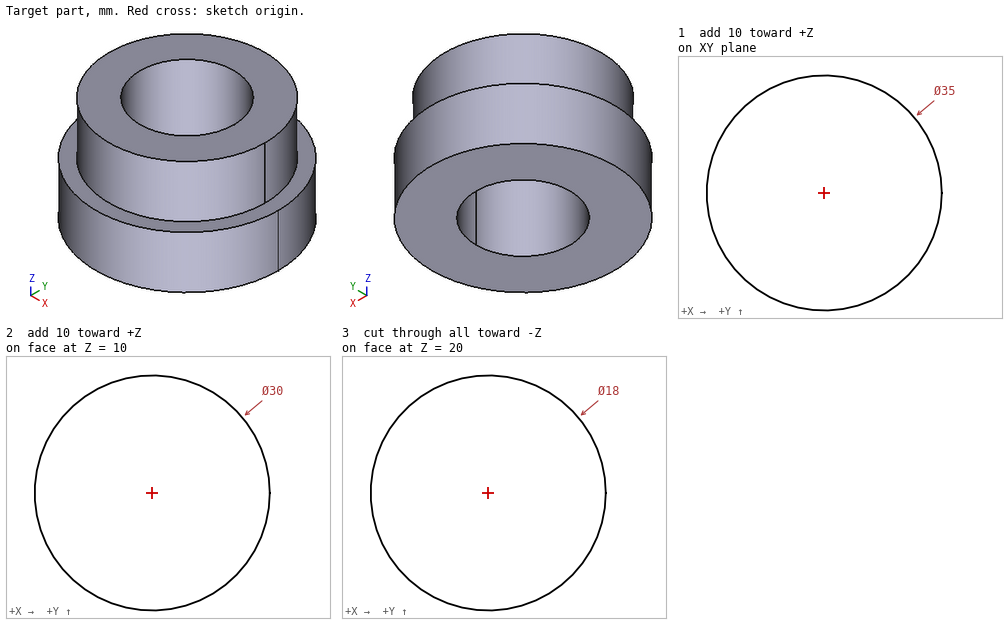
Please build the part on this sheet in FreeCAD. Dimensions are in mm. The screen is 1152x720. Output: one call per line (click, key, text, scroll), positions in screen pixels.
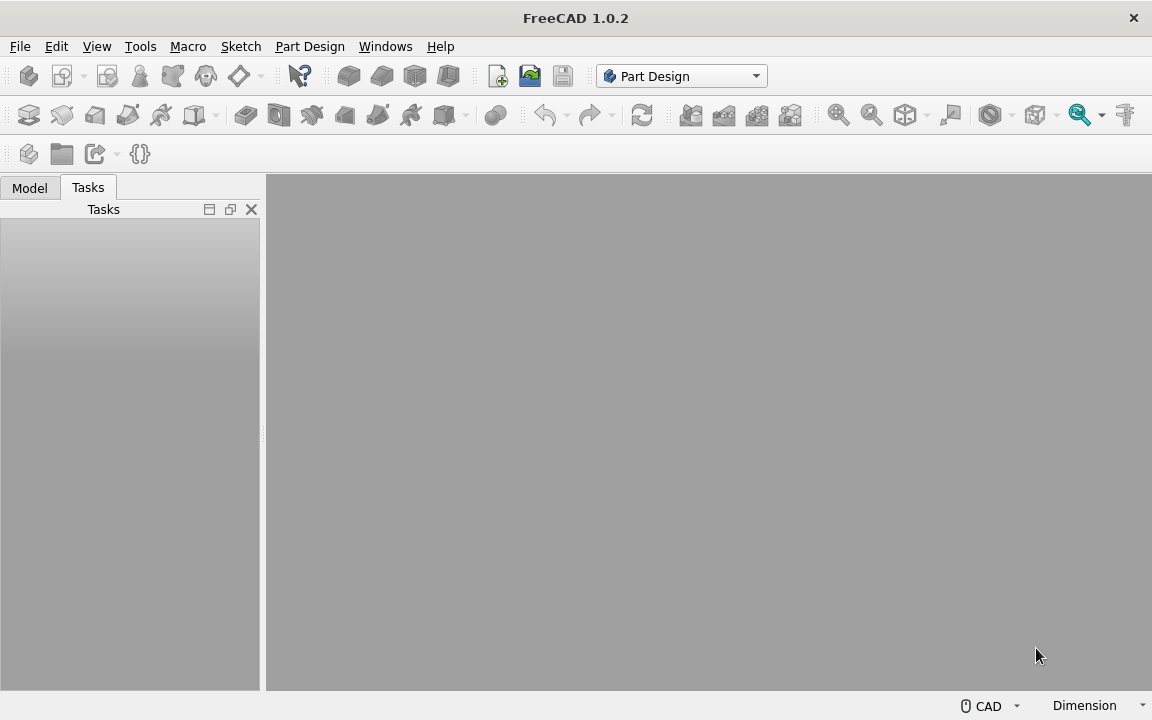
click(497, 76)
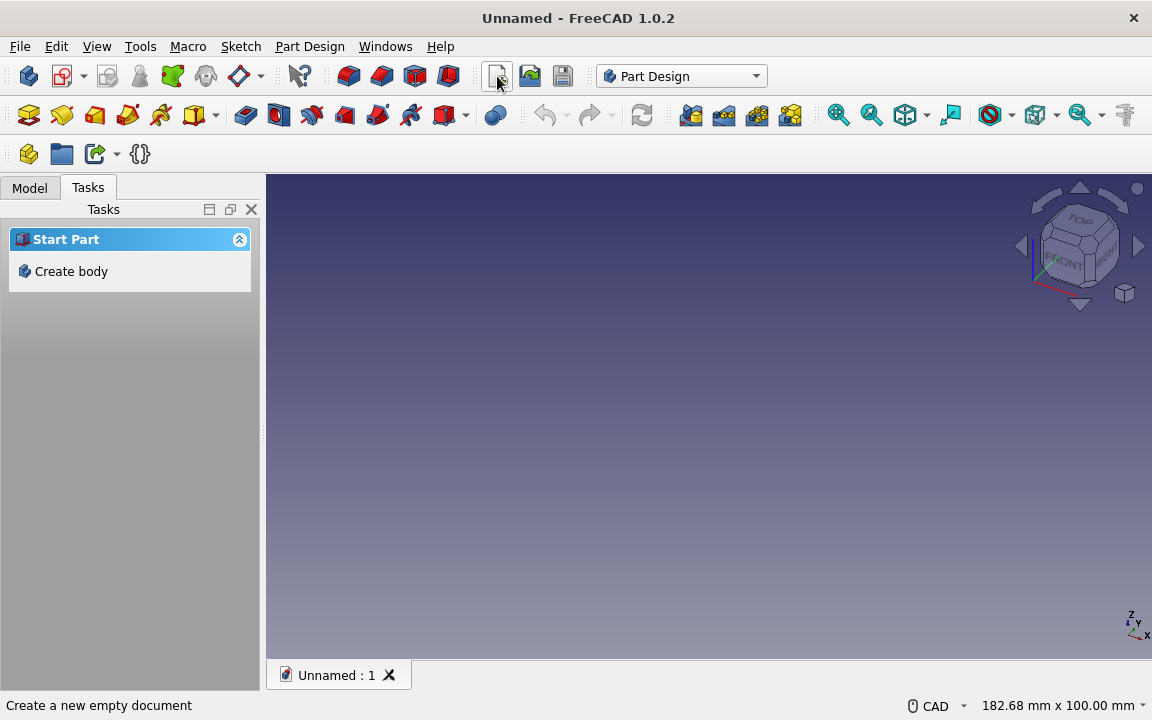
click(62, 76)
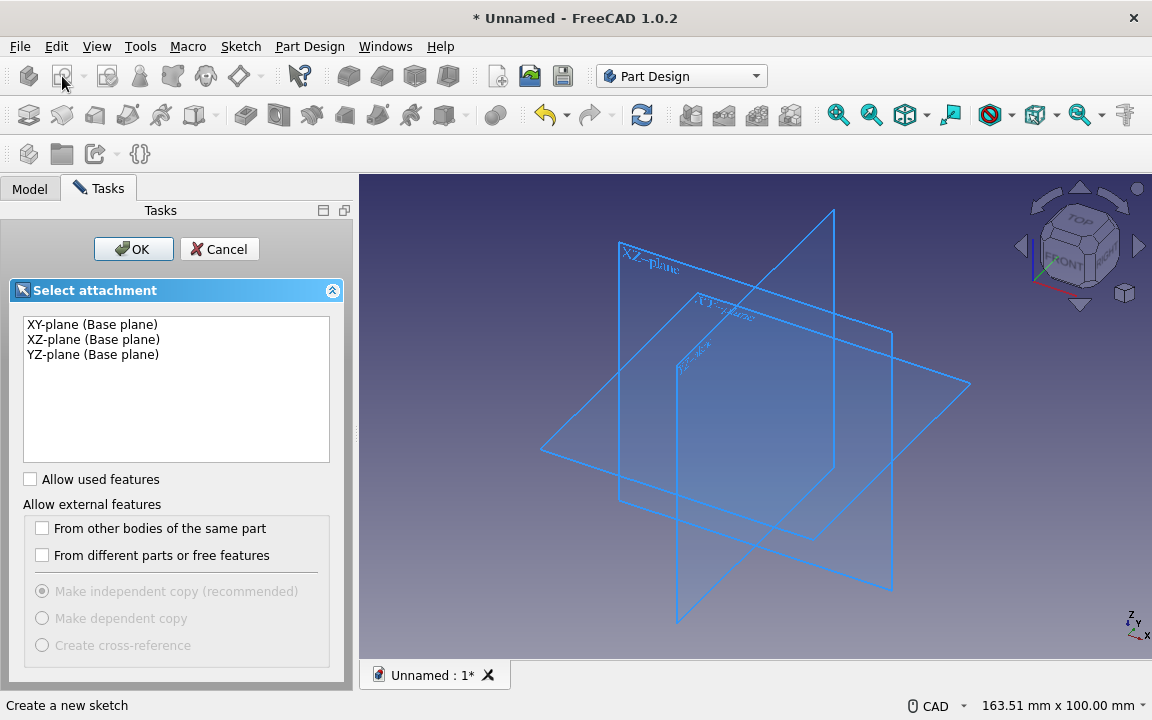
click(84, 324)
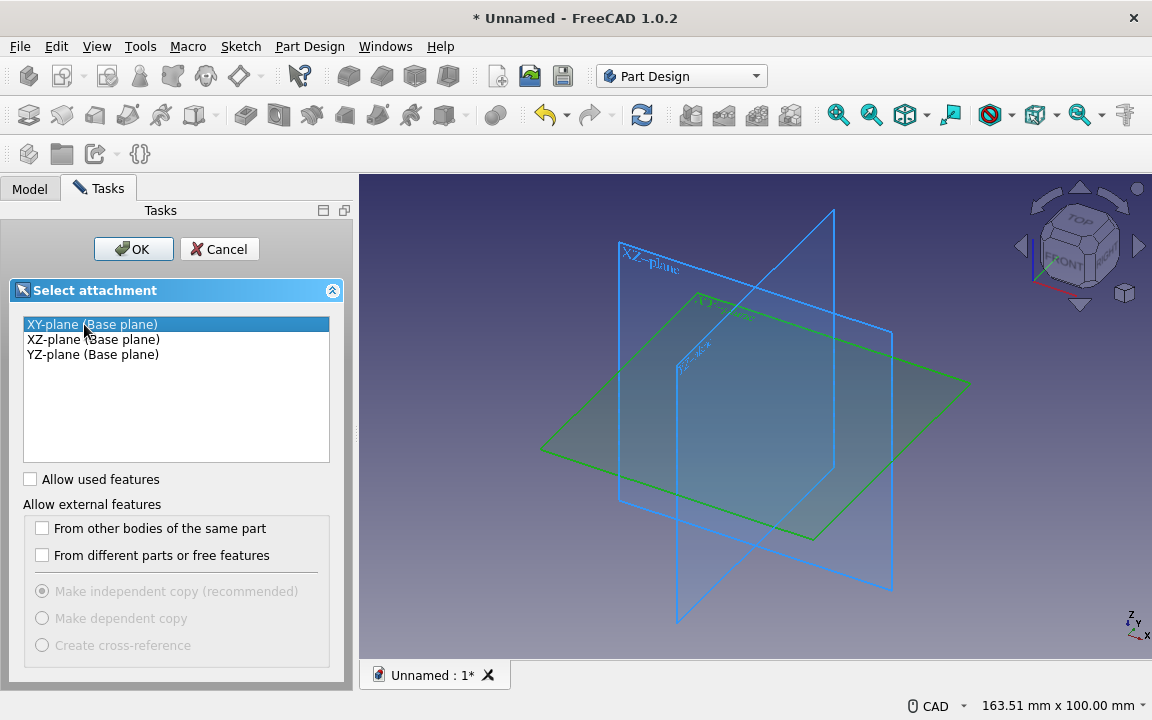
click(134, 249)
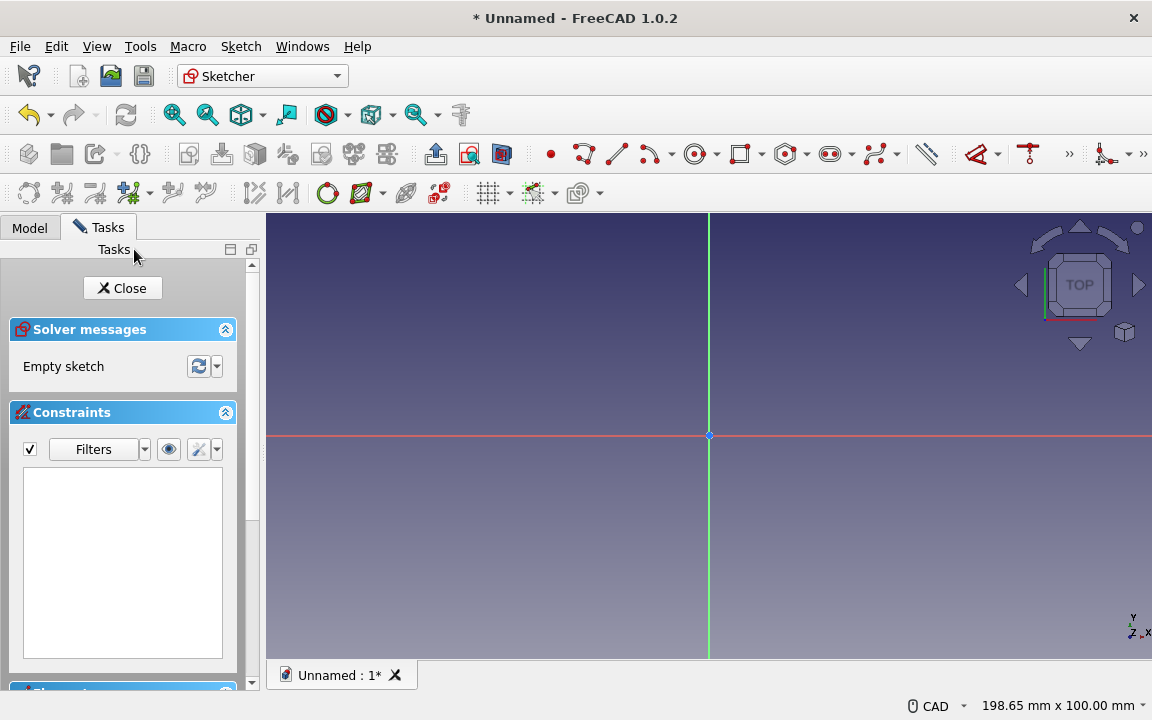
scroll(792, 436, up, 3)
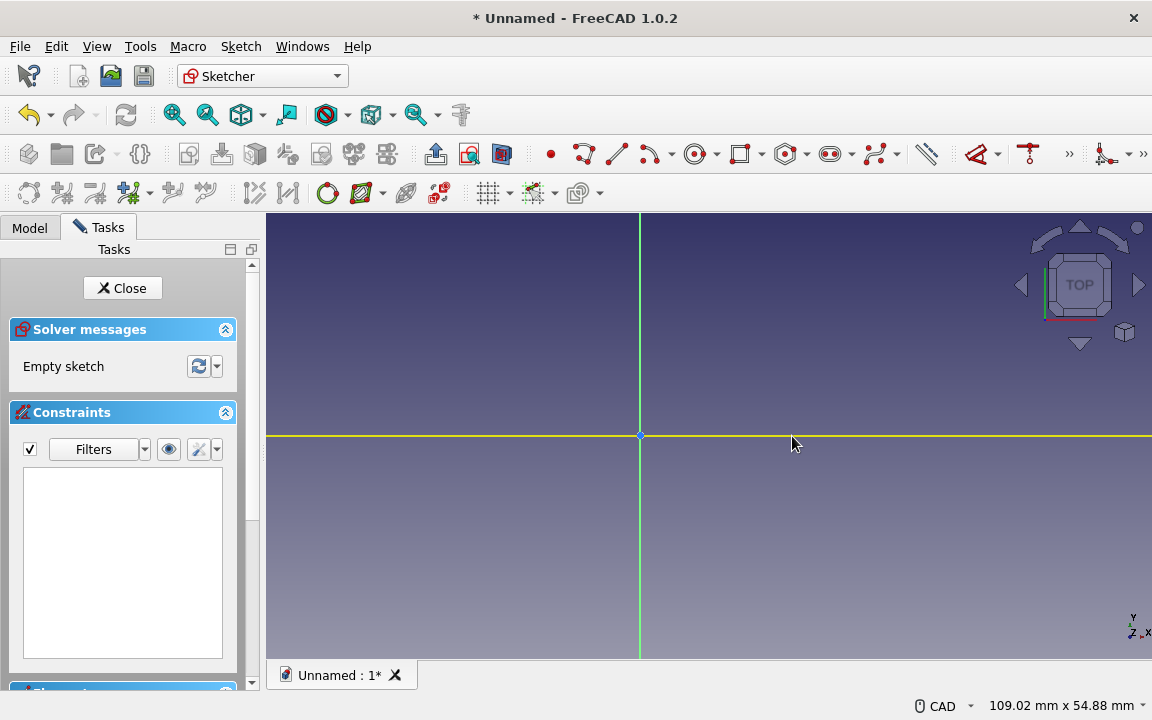
click(694, 154)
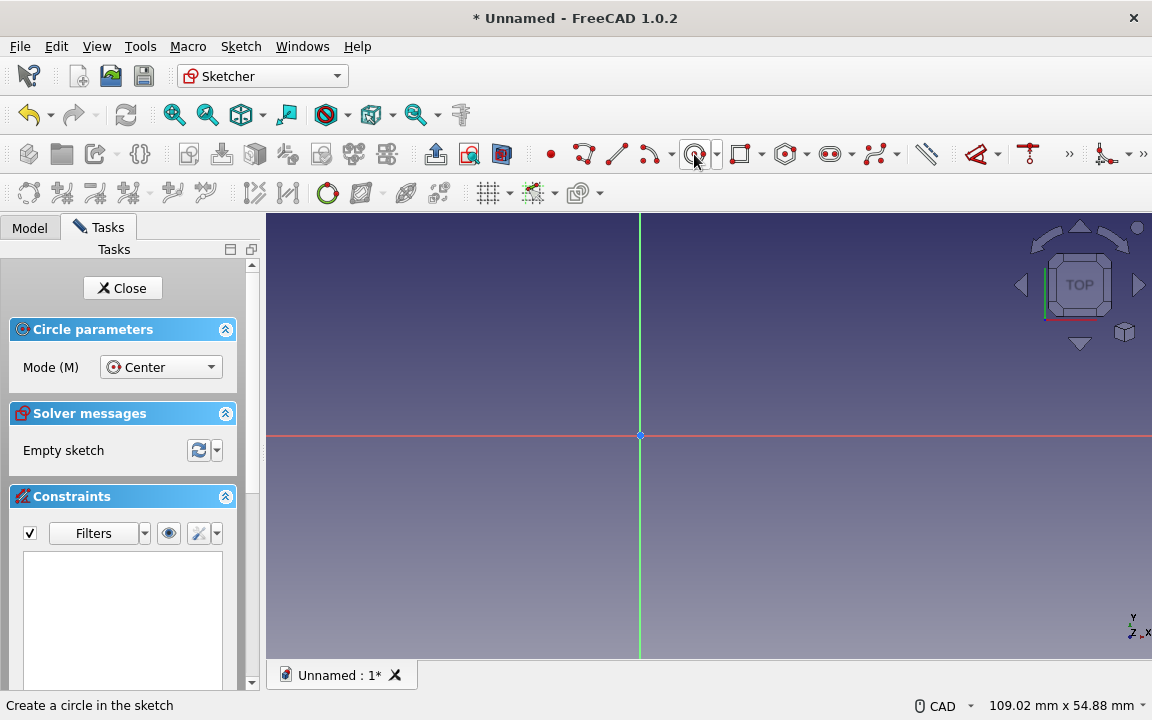
click(640, 436)
move(741, 335)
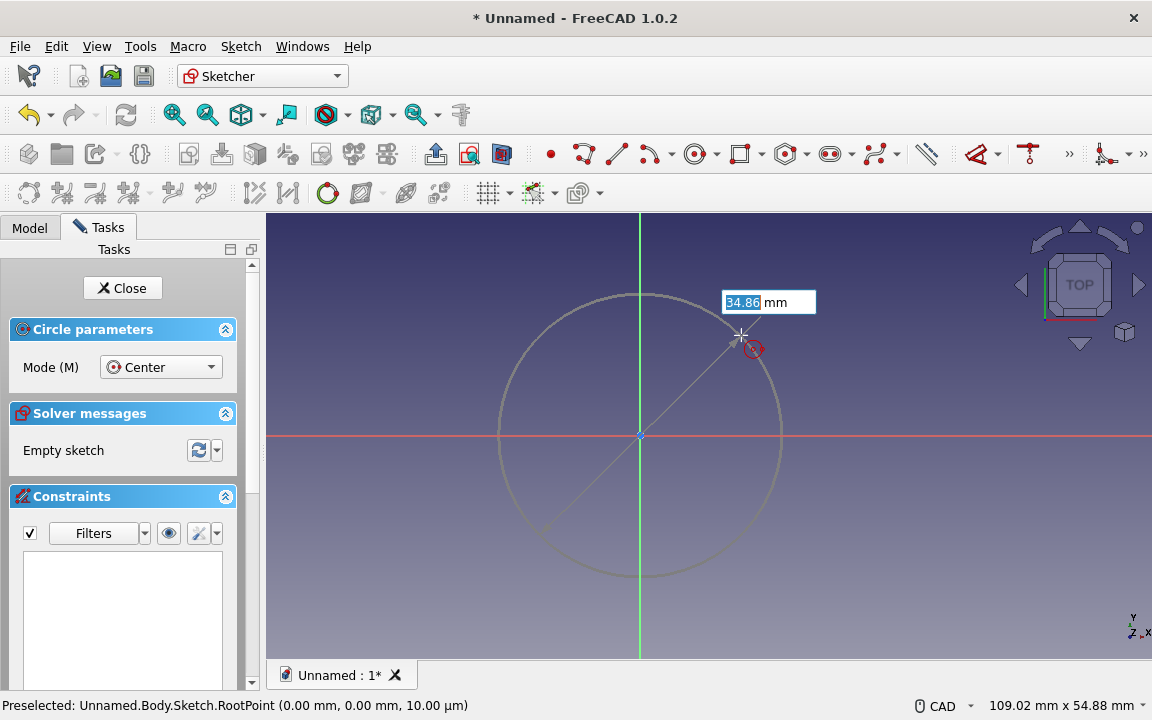
text(35)
key(Return)
key(Escape)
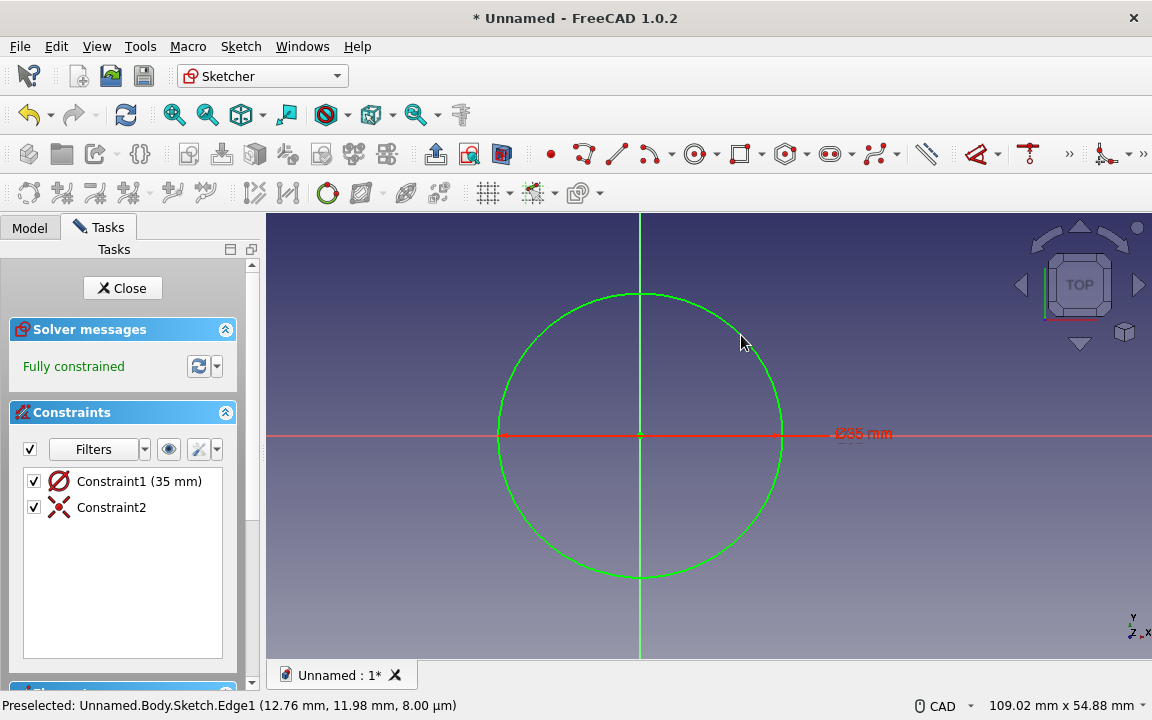
click(123, 288)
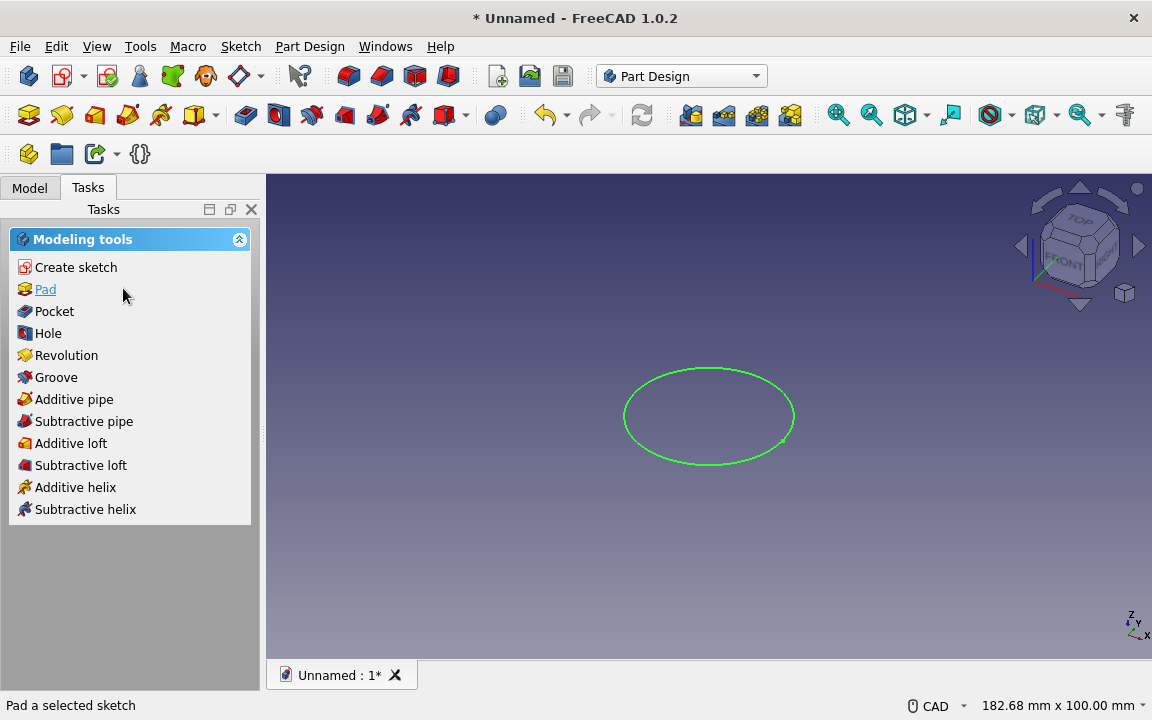
click(29, 116)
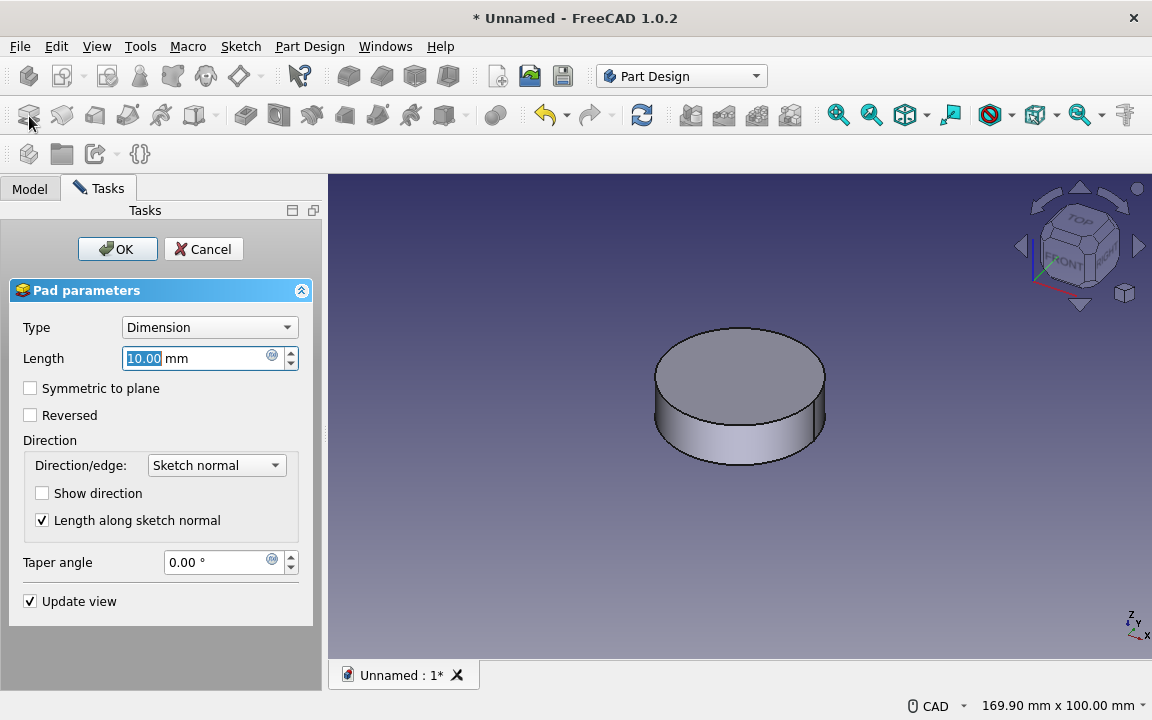
text(10)
key(Tab)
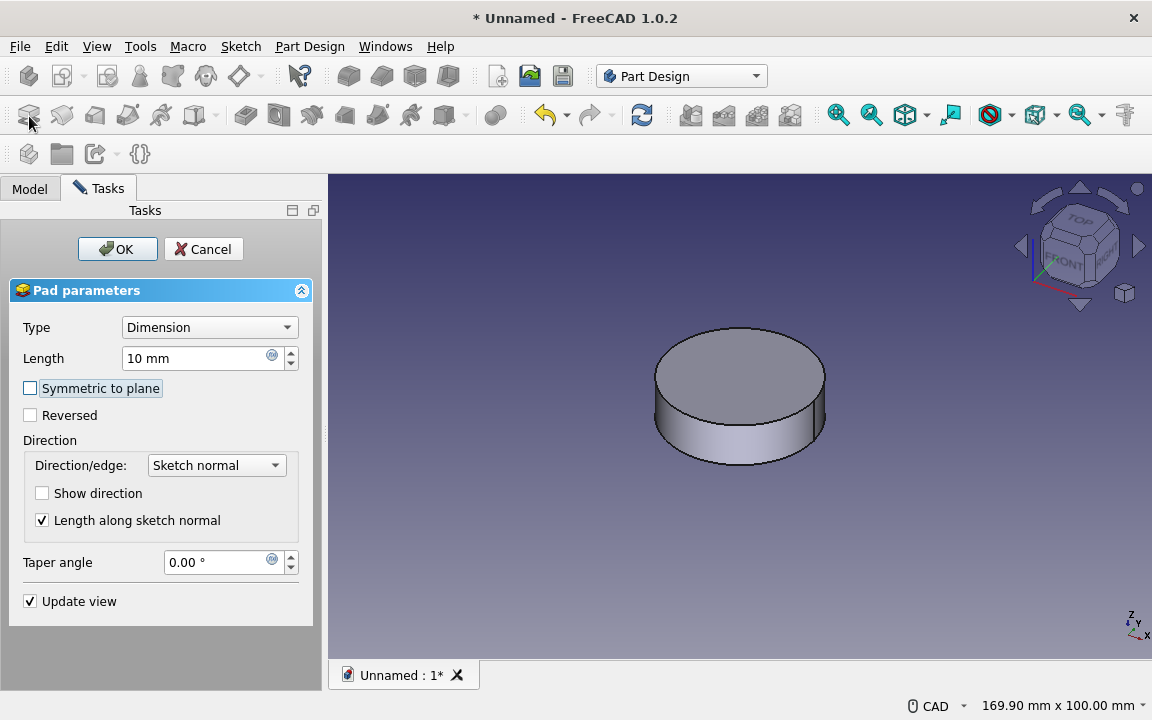
click(118, 249)